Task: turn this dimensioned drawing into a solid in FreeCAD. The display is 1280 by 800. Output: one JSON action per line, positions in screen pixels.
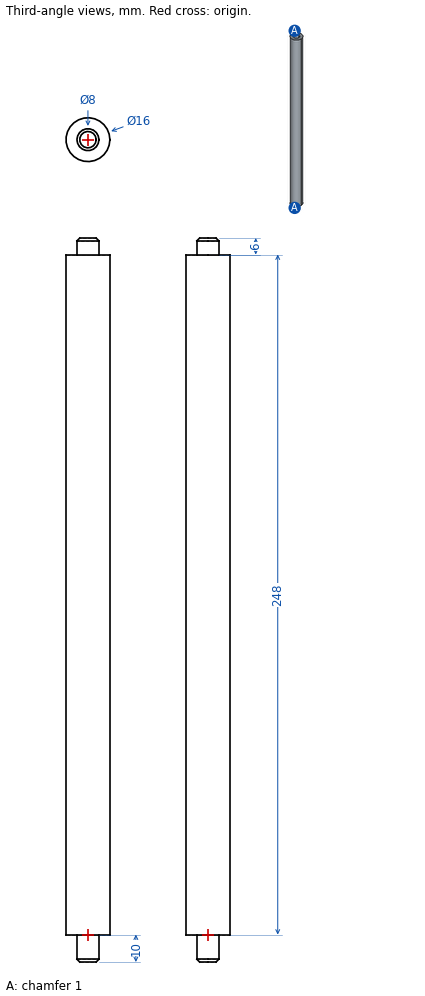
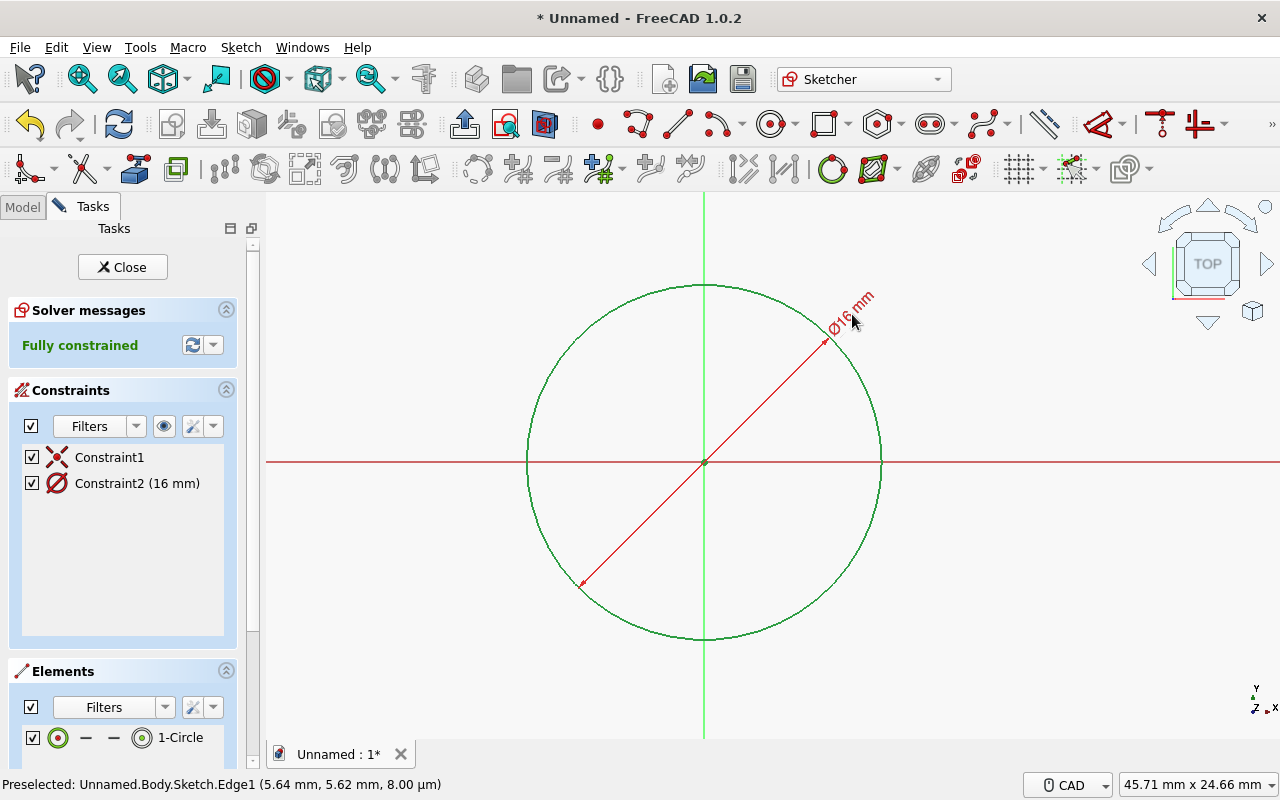
{"action": "left_click", "coordinate": [123, 267]}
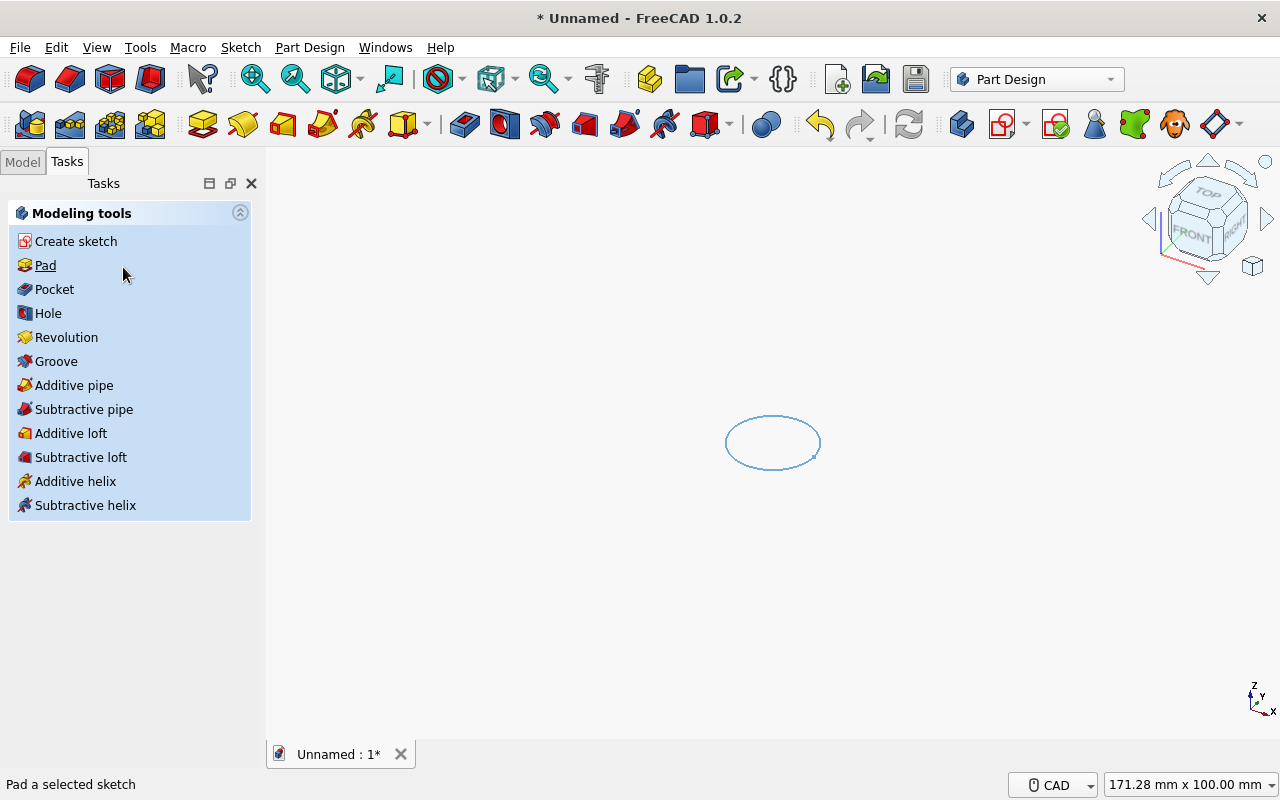
{"action": "left_click", "coordinate": [204, 124]}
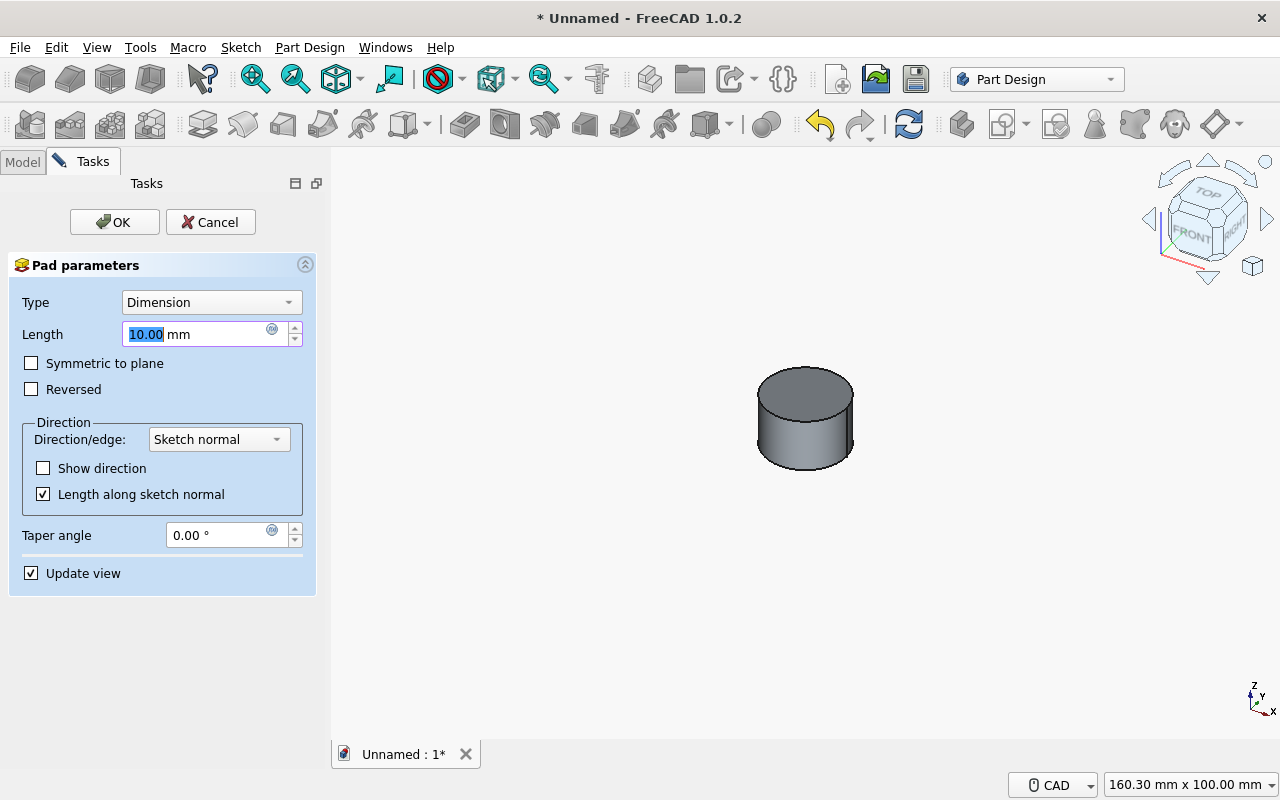
{"action": "type", "text": "248"}
{"action": "key", "text": "Tab"}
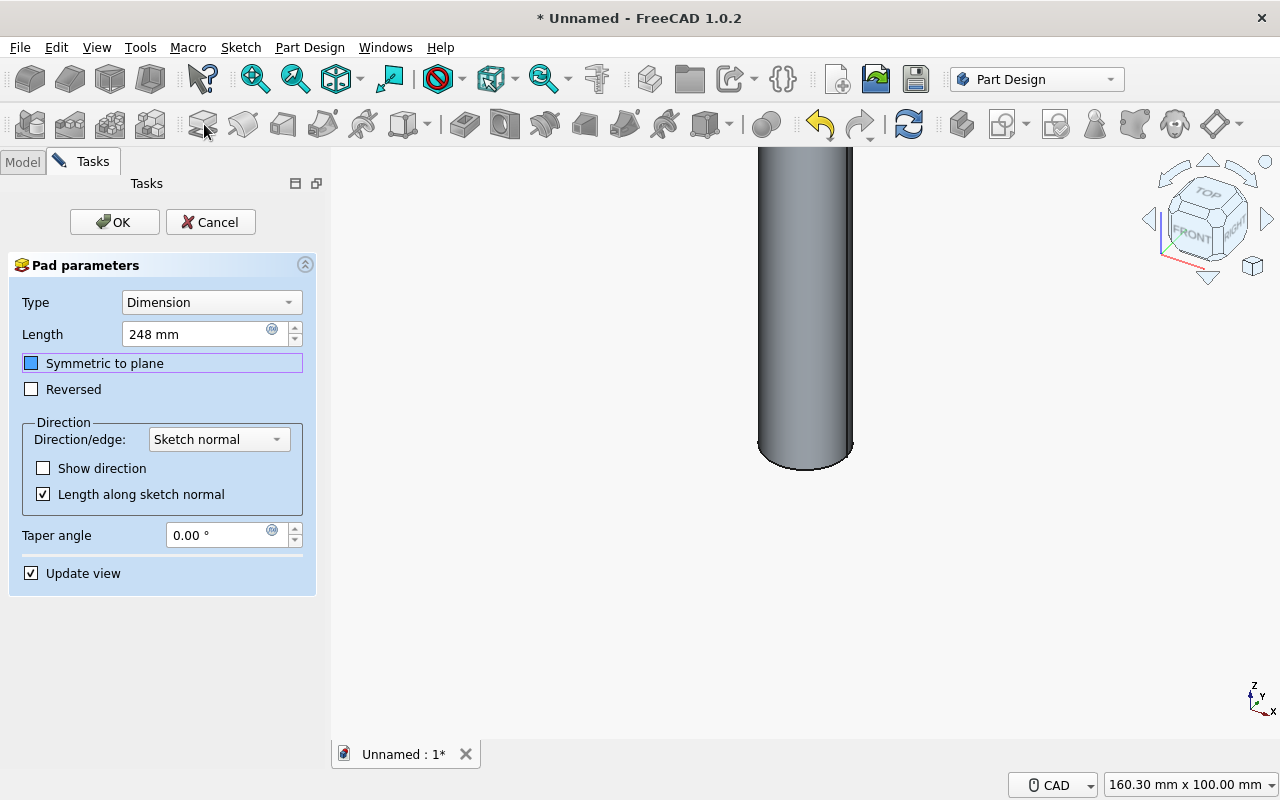
{"action": "left_click", "coordinate": [115, 222]}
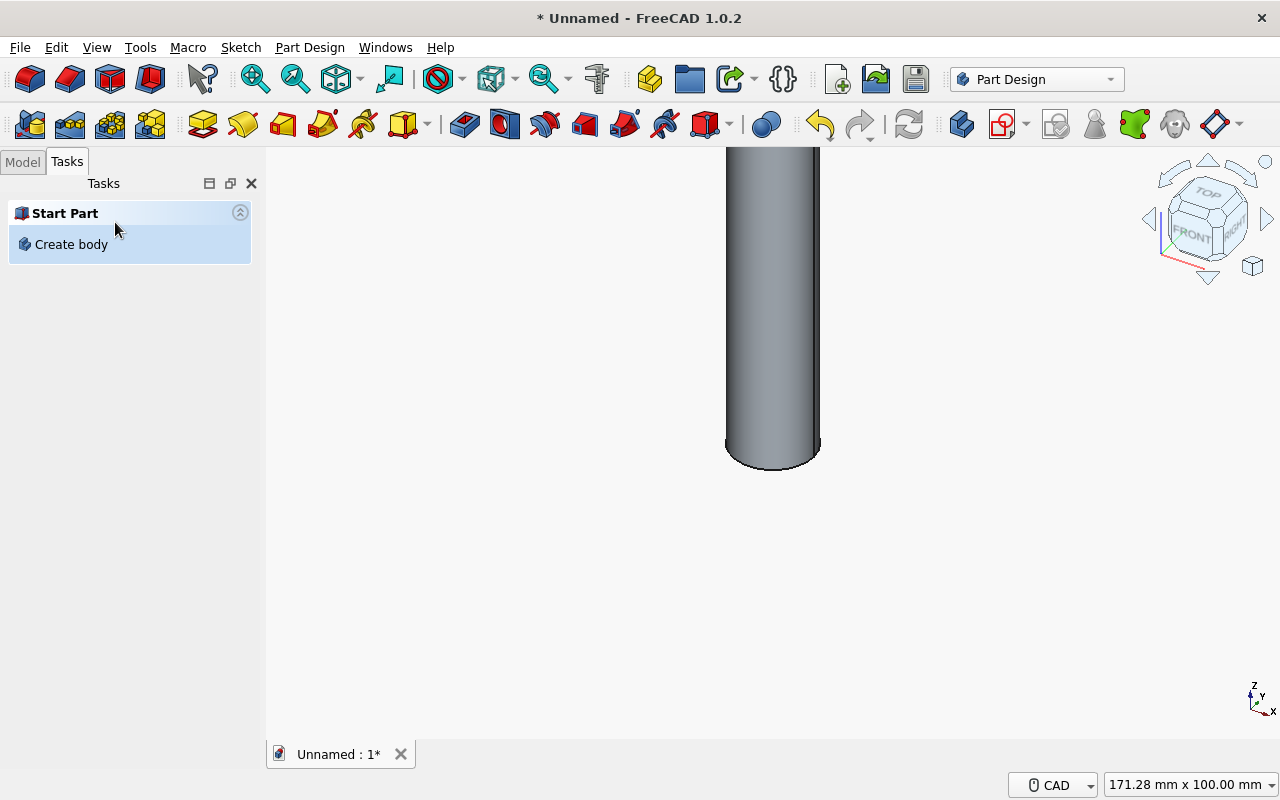
{"action": "key", "text": "v f"}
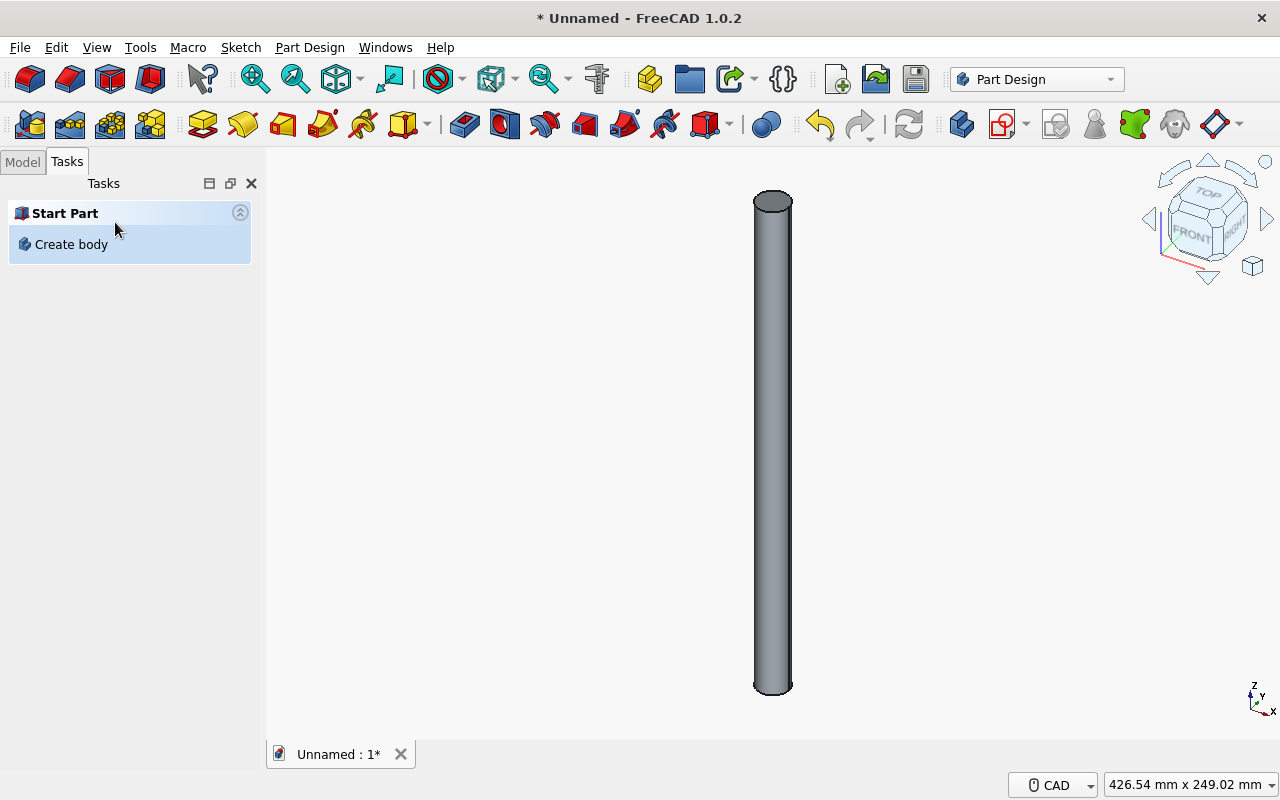
{"action": "left_click", "coordinate": [1002, 124]}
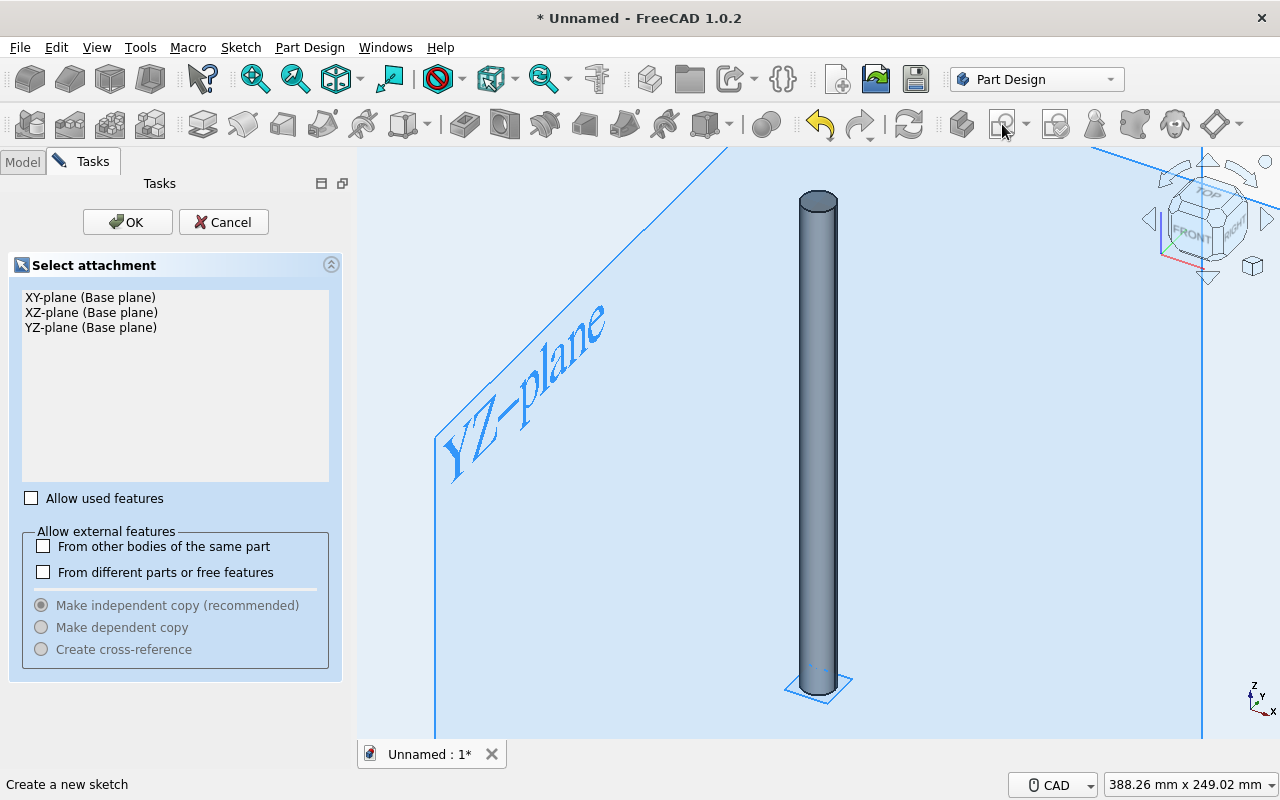
{"action": "left_click", "coordinate": [82, 298]}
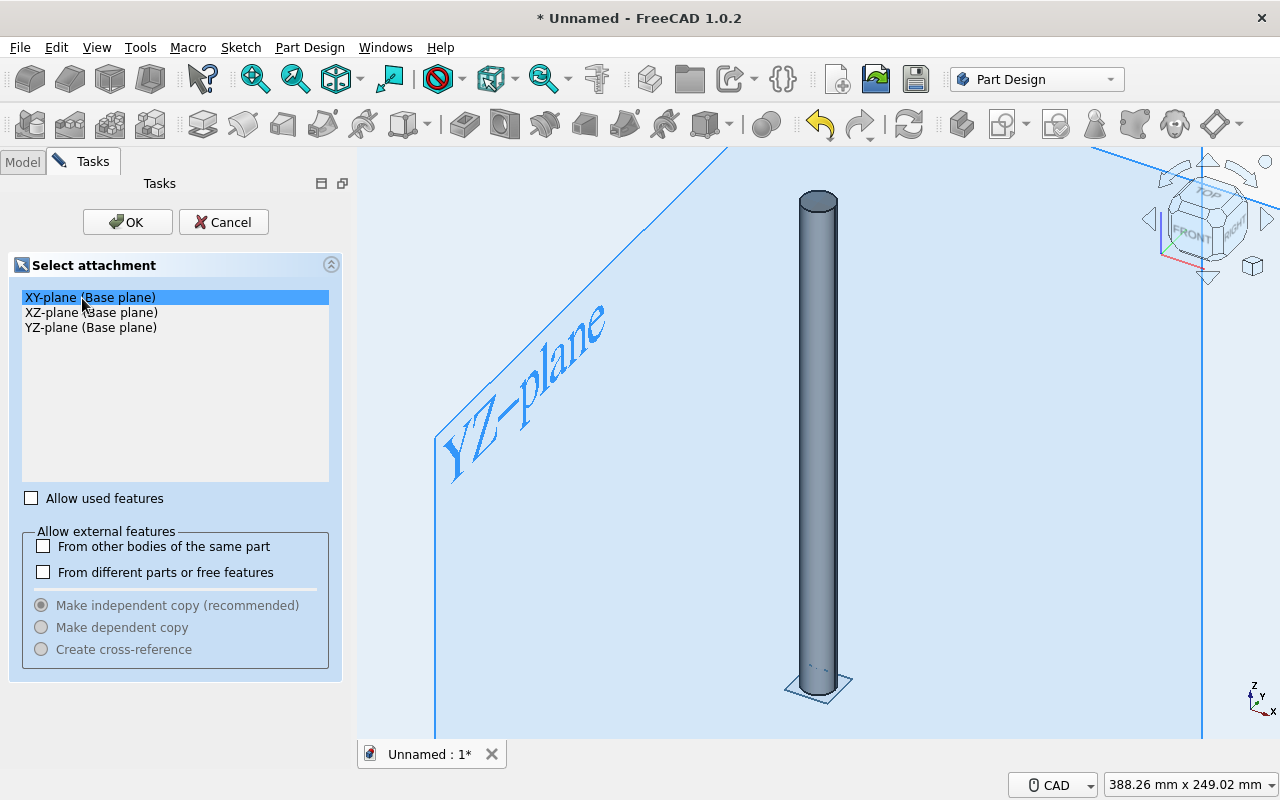
{"action": "left_click", "coordinate": [128, 222]}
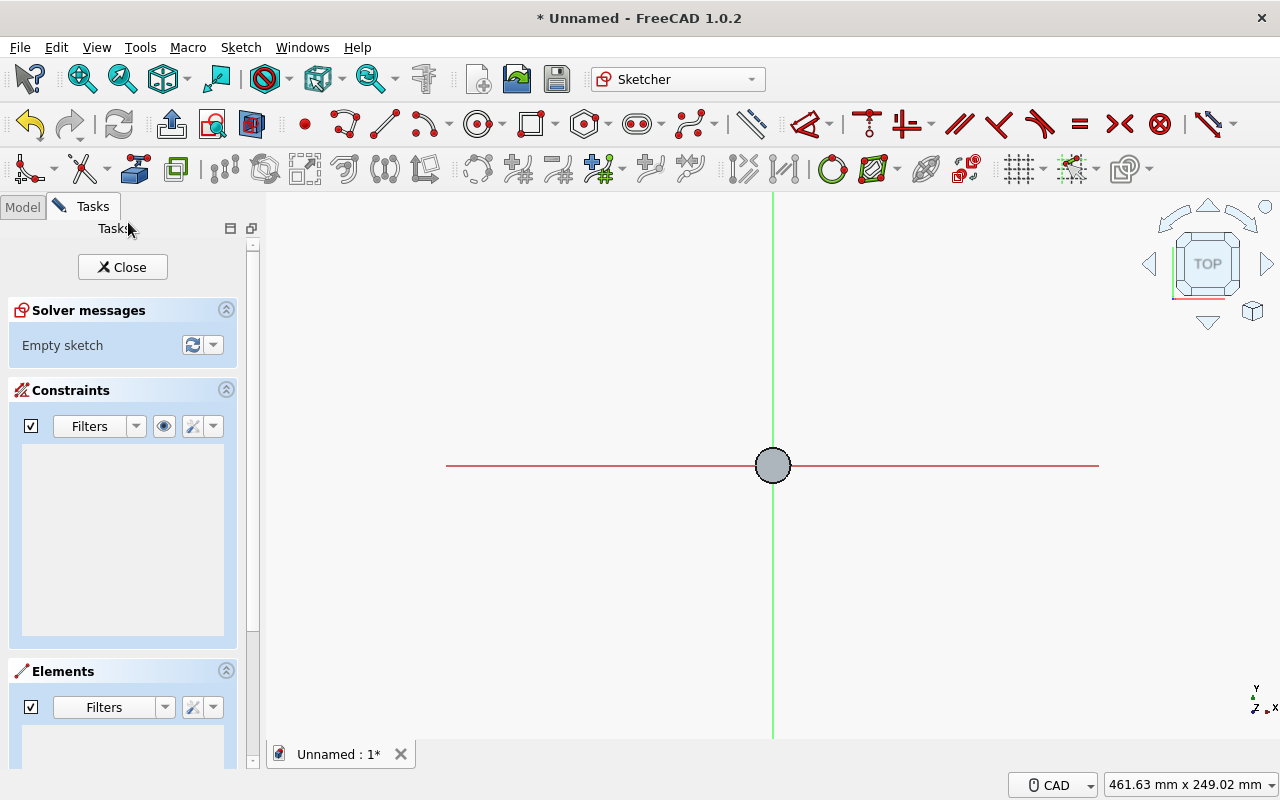
{"action": "key", "text": "q s"}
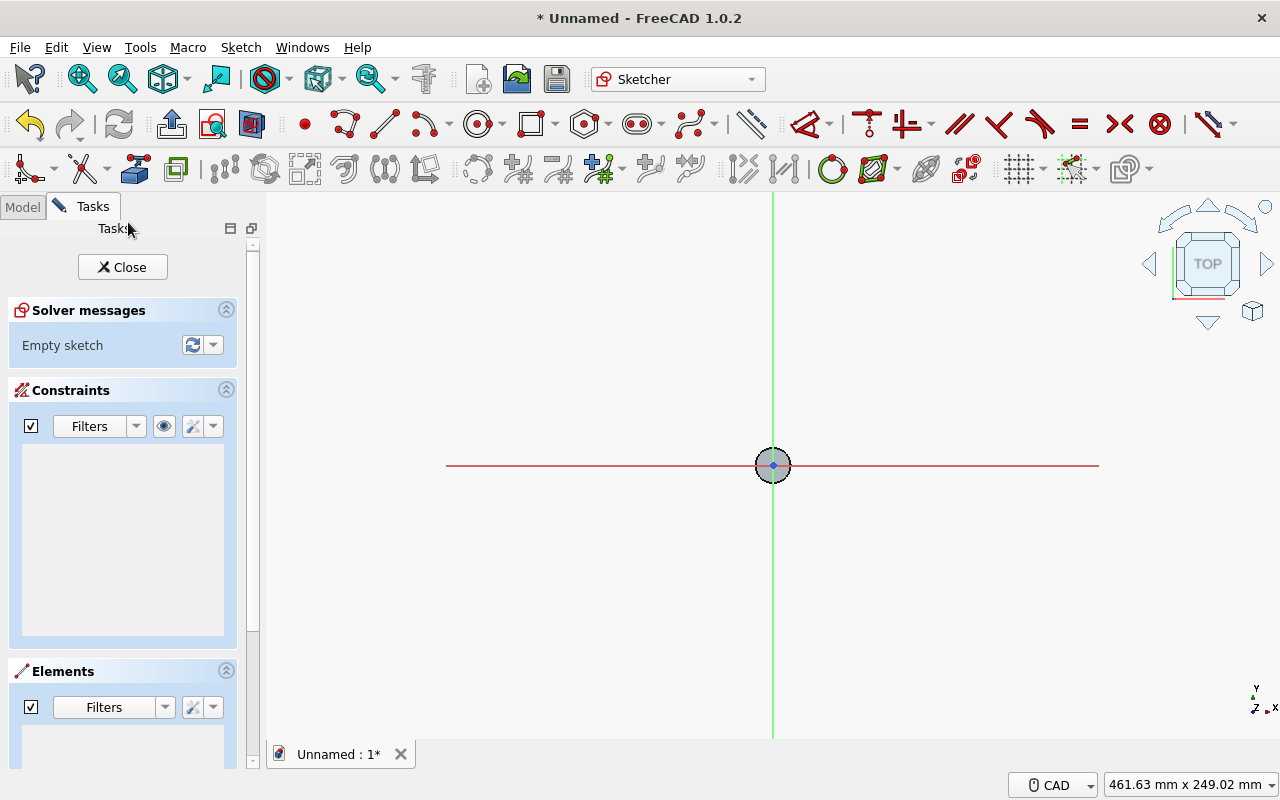
{"action": "scroll", "coordinate": [777, 466], "scroll_direction": "up", "scroll_amount": 15}